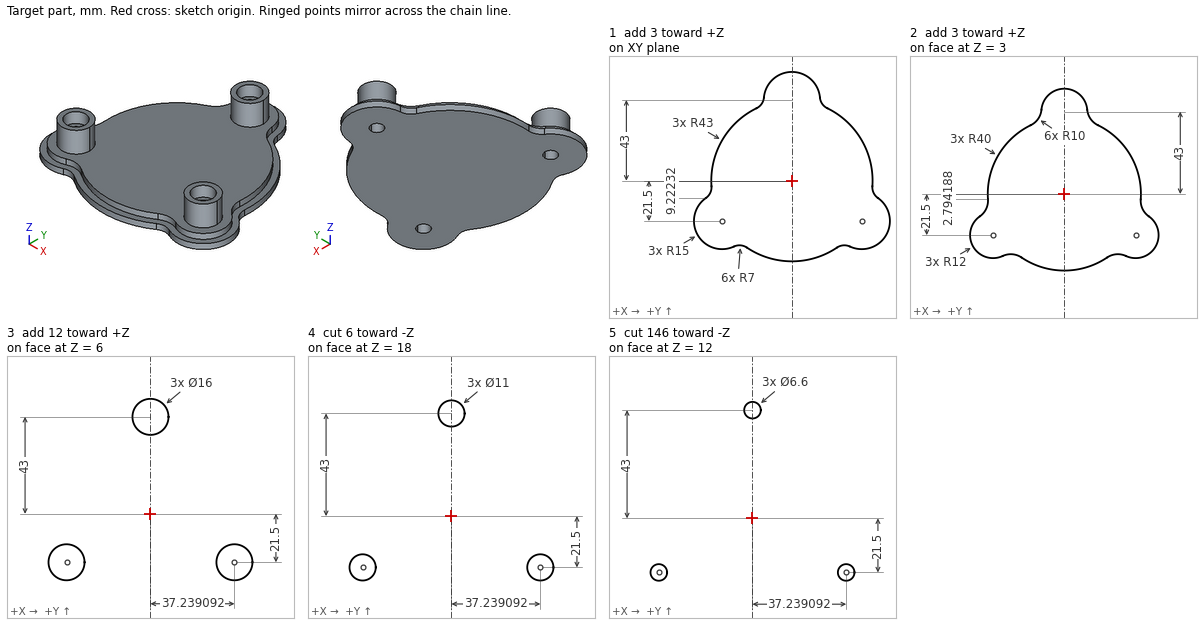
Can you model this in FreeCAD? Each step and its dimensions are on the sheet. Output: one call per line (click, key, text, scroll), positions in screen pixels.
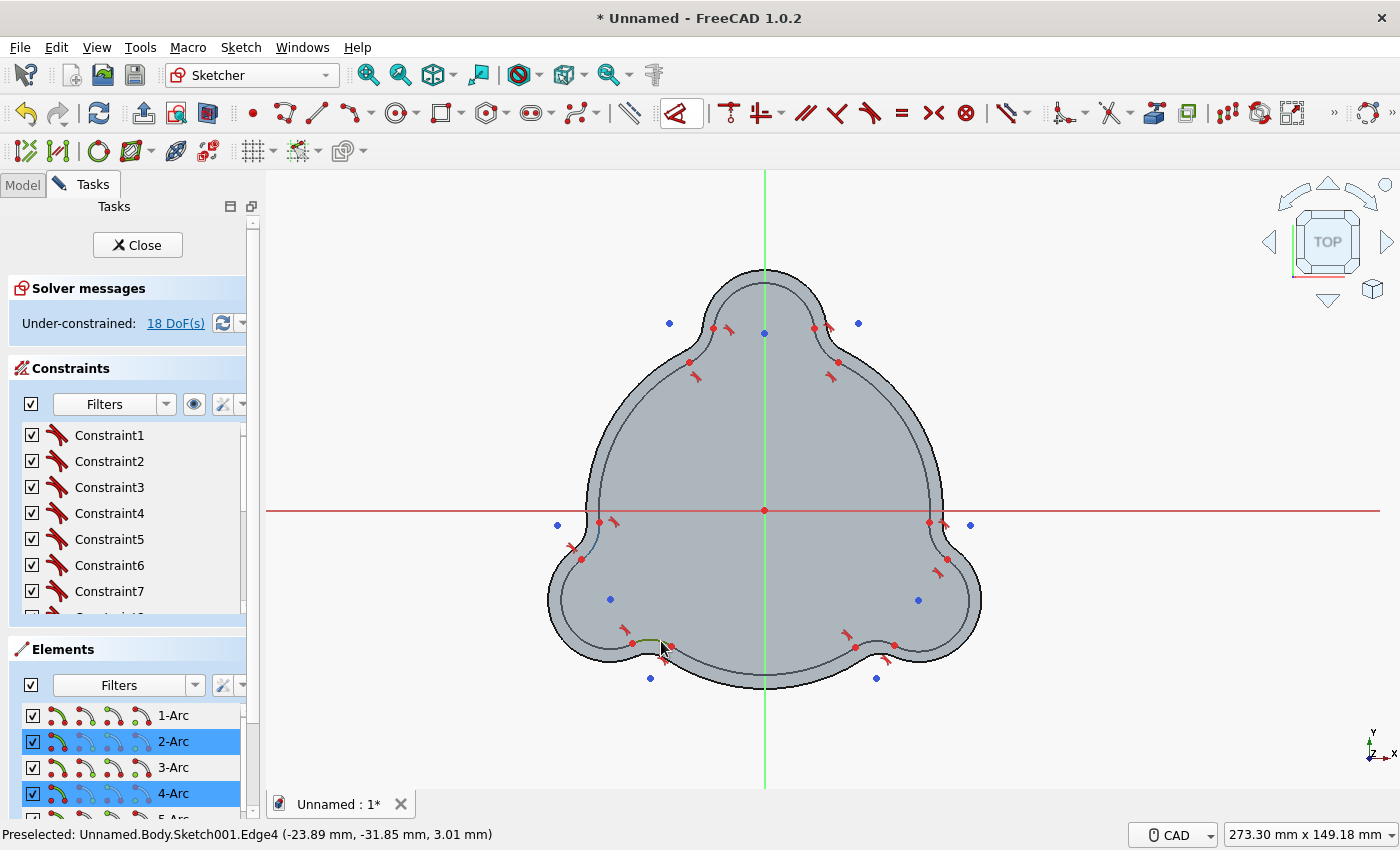
click(883, 642)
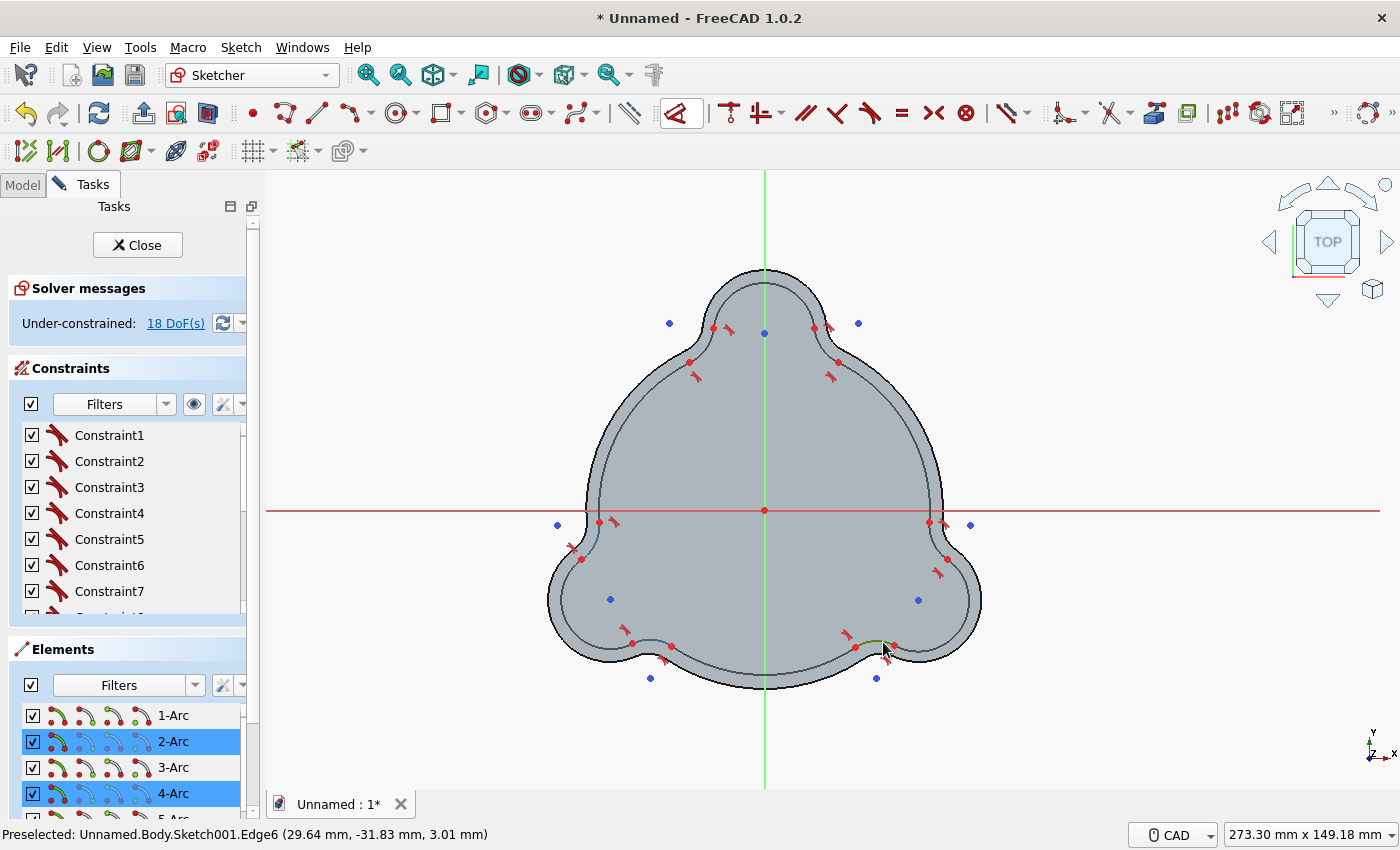
click(931, 535)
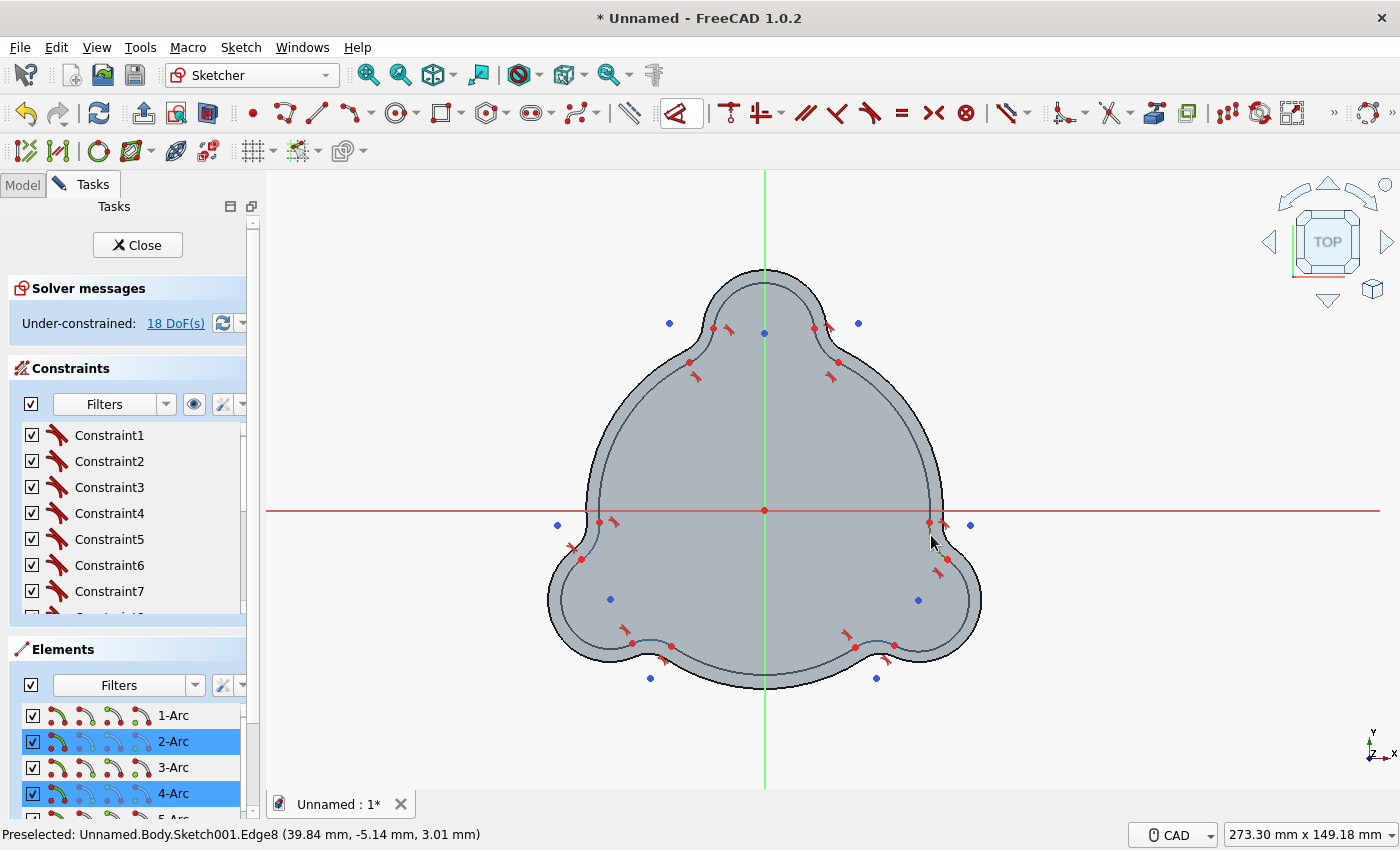
click(818, 341)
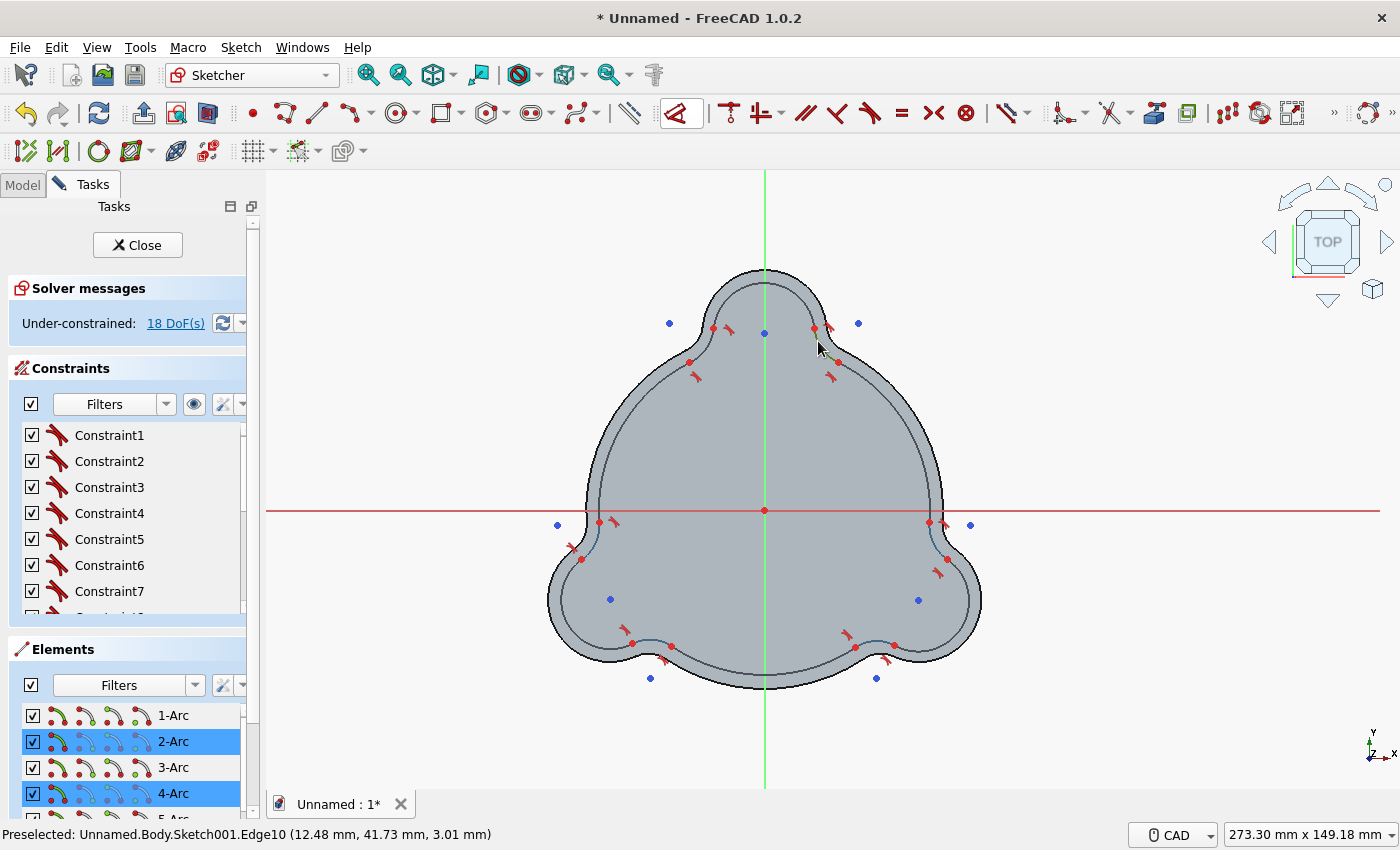
click(701, 355)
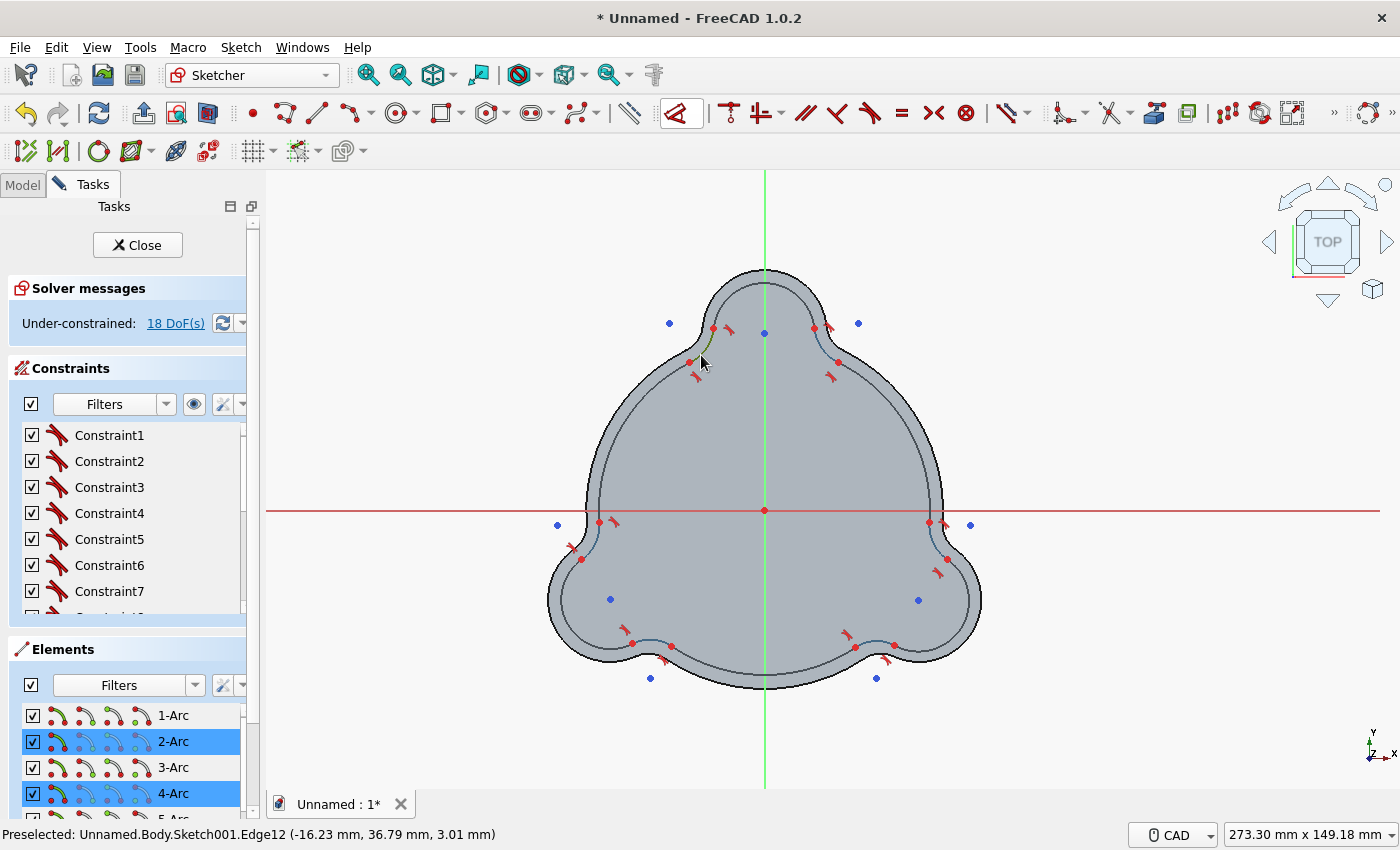
click(902, 114)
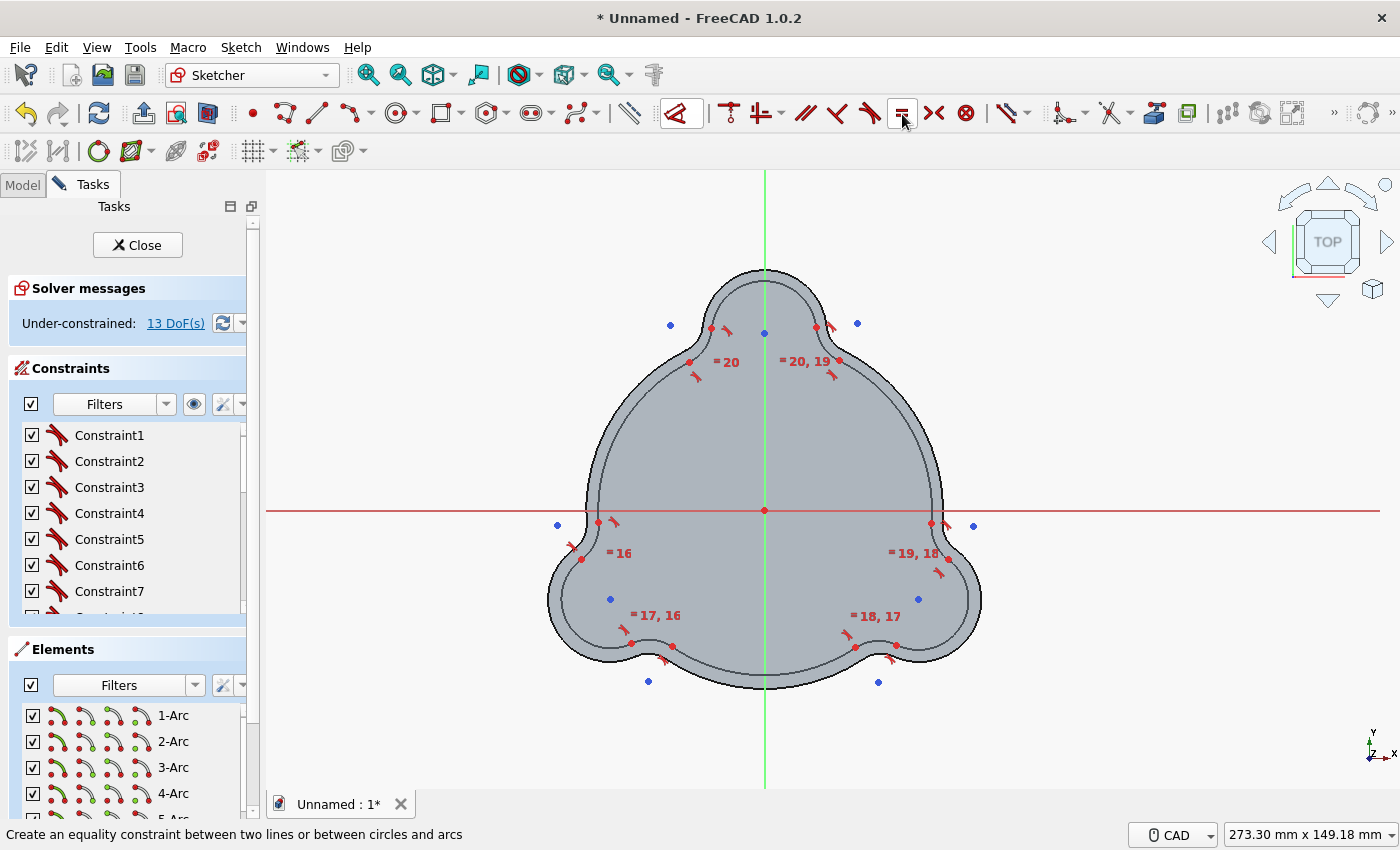
click(643, 397)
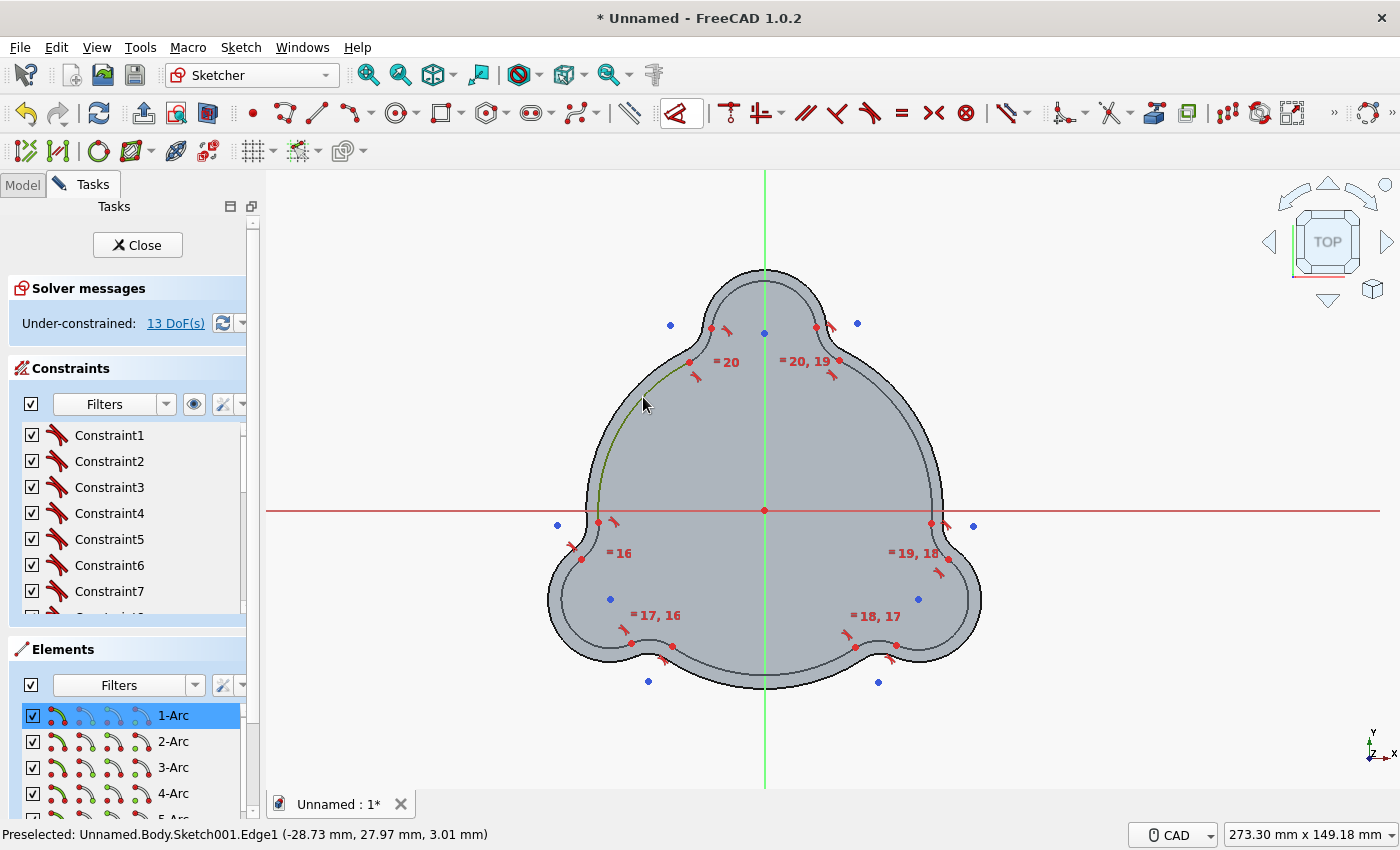
click(725, 670)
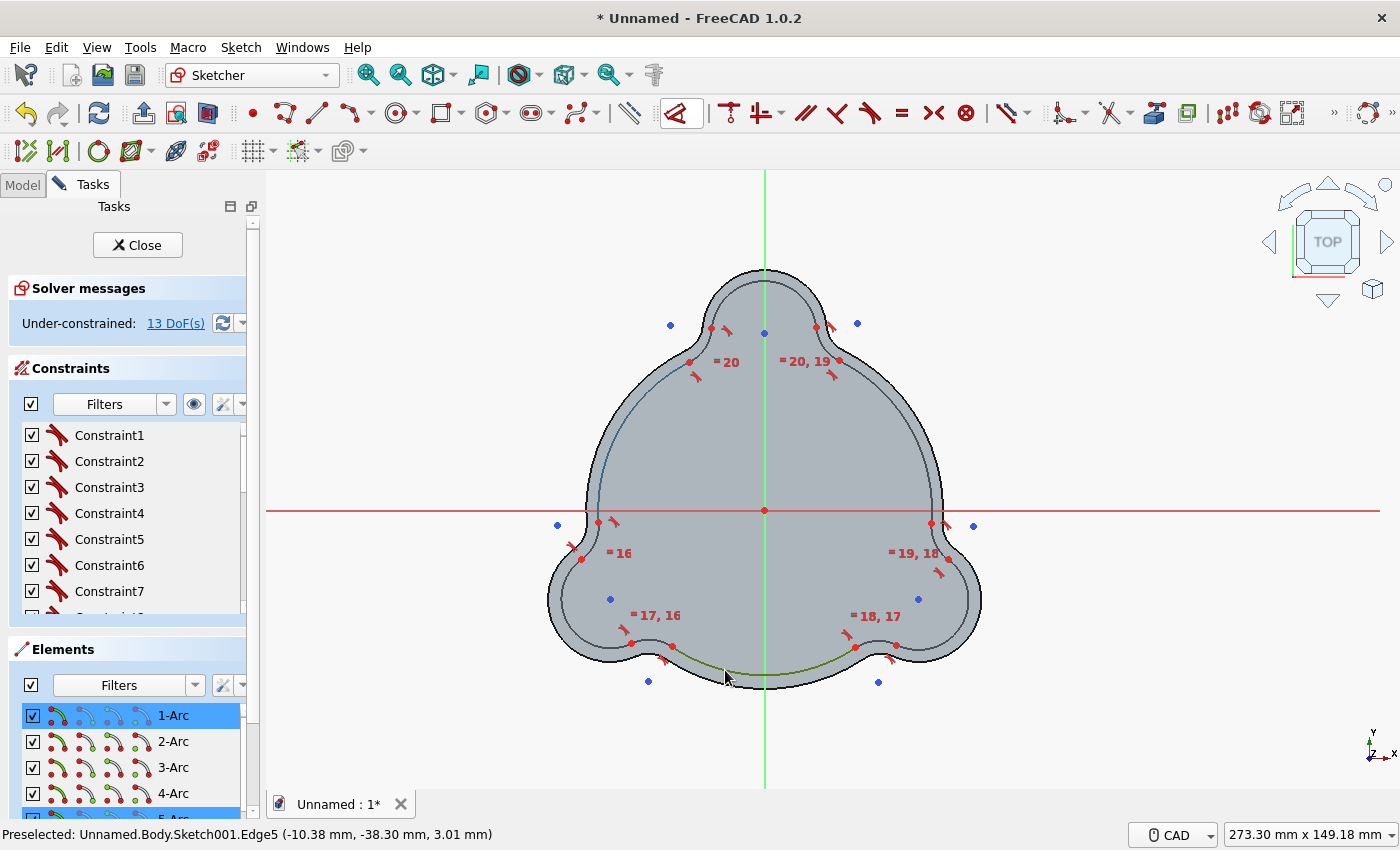
click(925, 464)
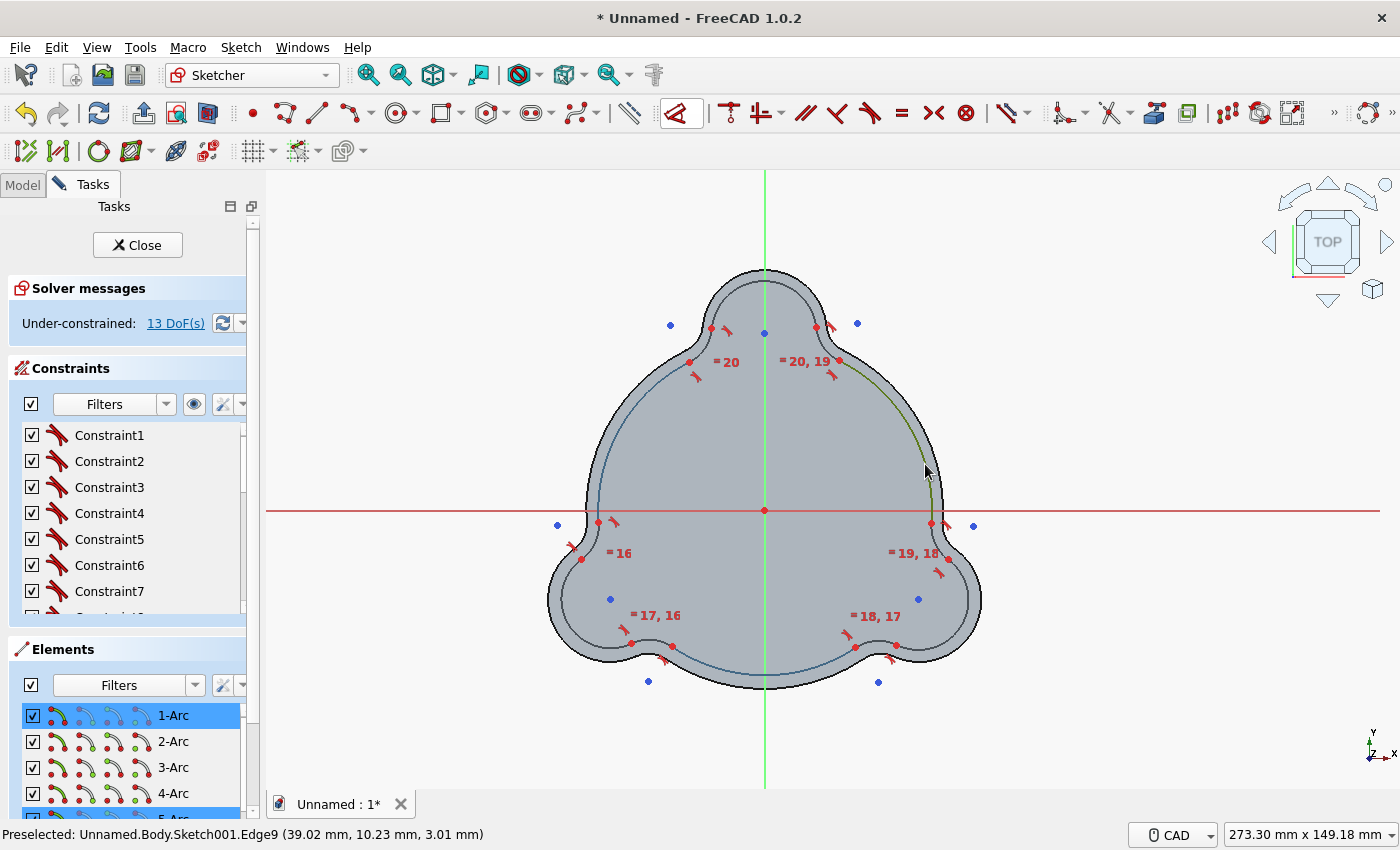
click(902, 114)